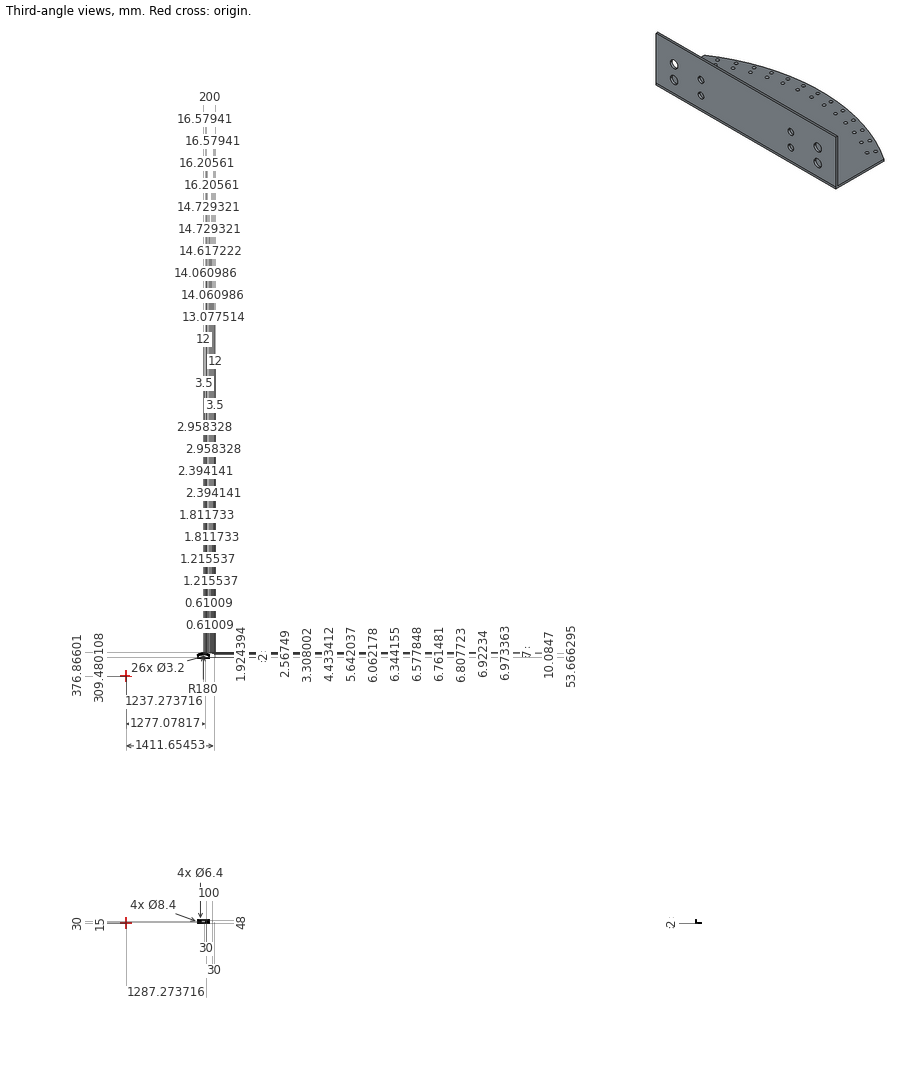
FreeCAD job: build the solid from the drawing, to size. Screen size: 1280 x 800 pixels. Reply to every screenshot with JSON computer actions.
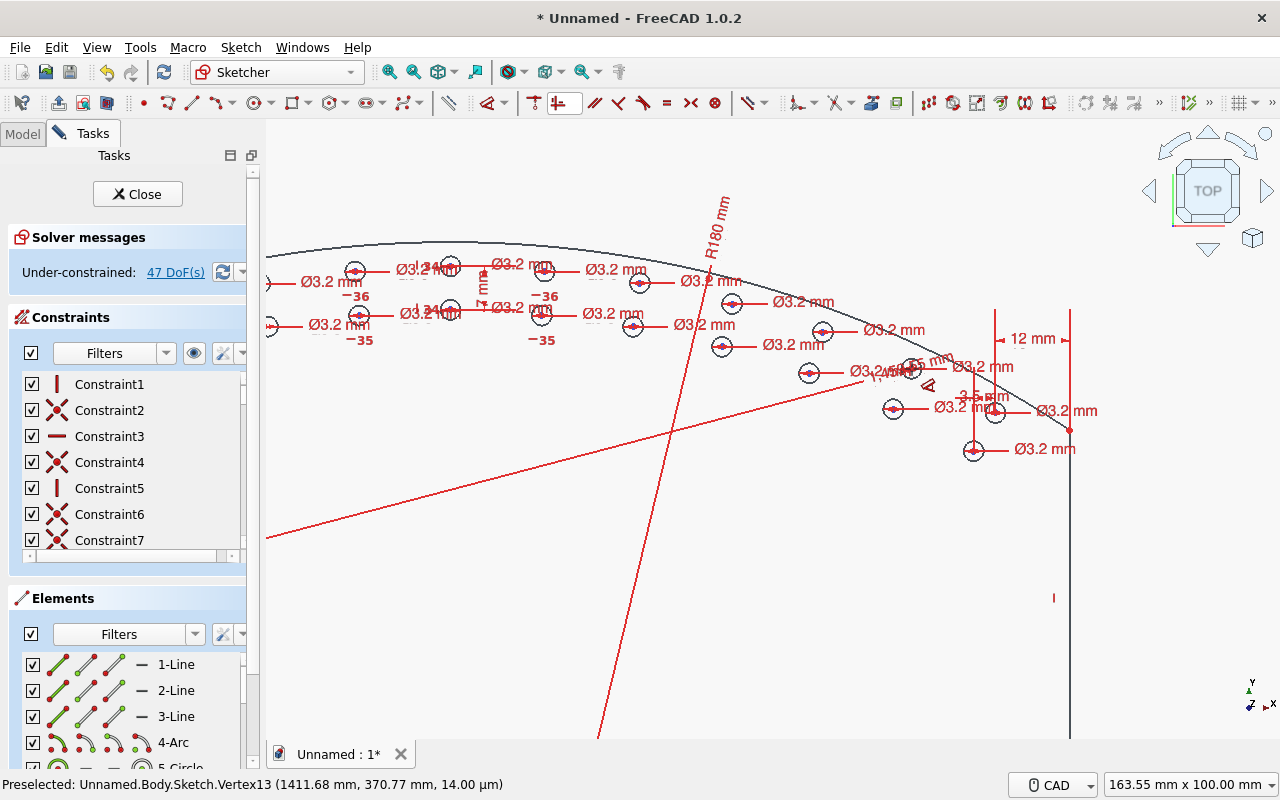
{"action": "left_click", "coordinate": [633, 327]}
{"action": "left_click", "coordinate": [946, 338]}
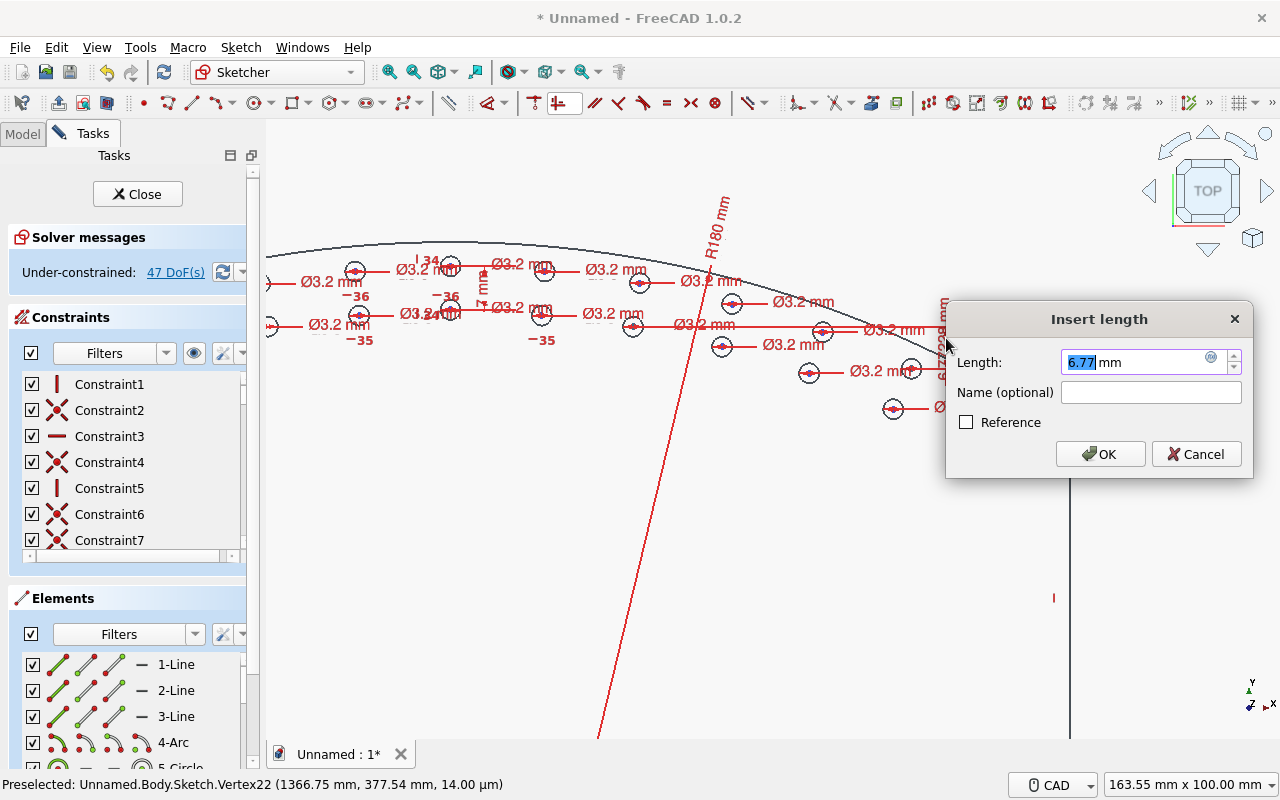
{"action": "type", "text": "6.92234"}
{"action": "key", "text": "Return"}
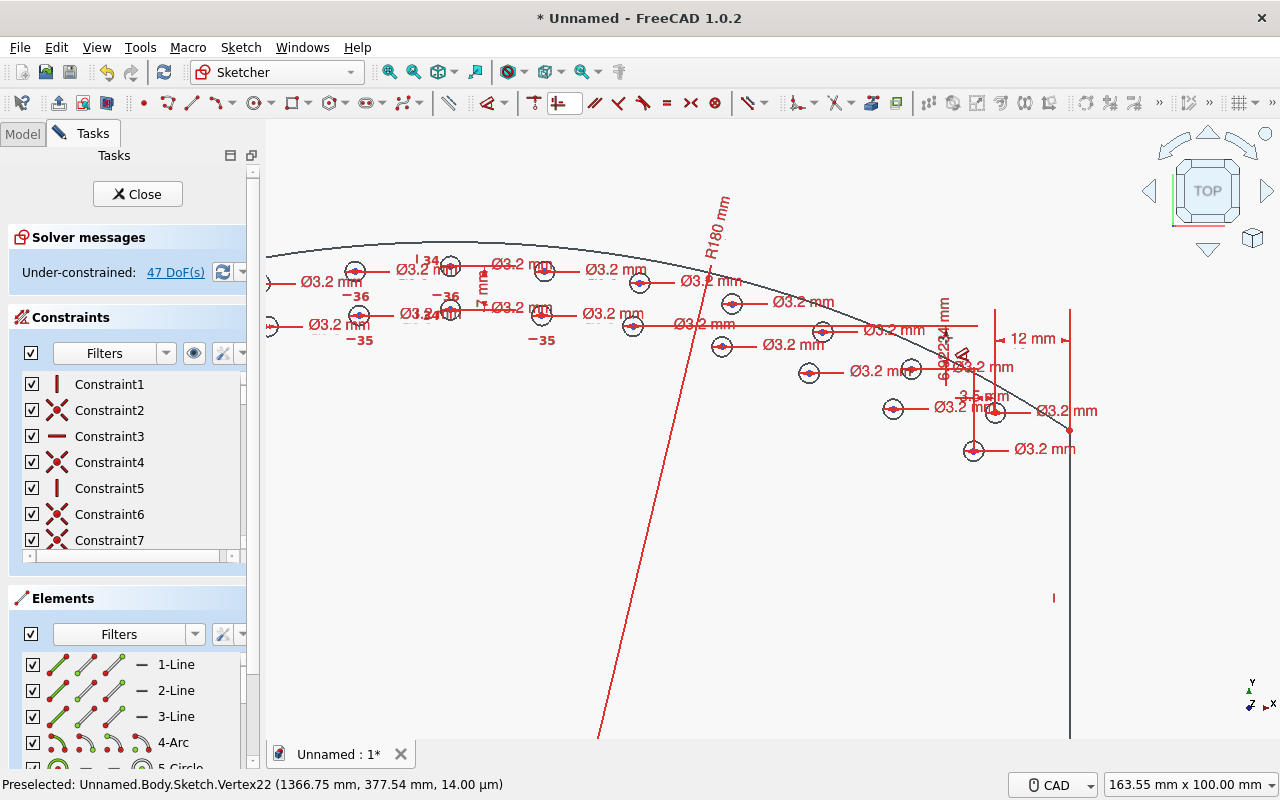
{"action": "scroll", "coordinate": [633, 326], "scroll_direction": "up", "scroll_amount": 5}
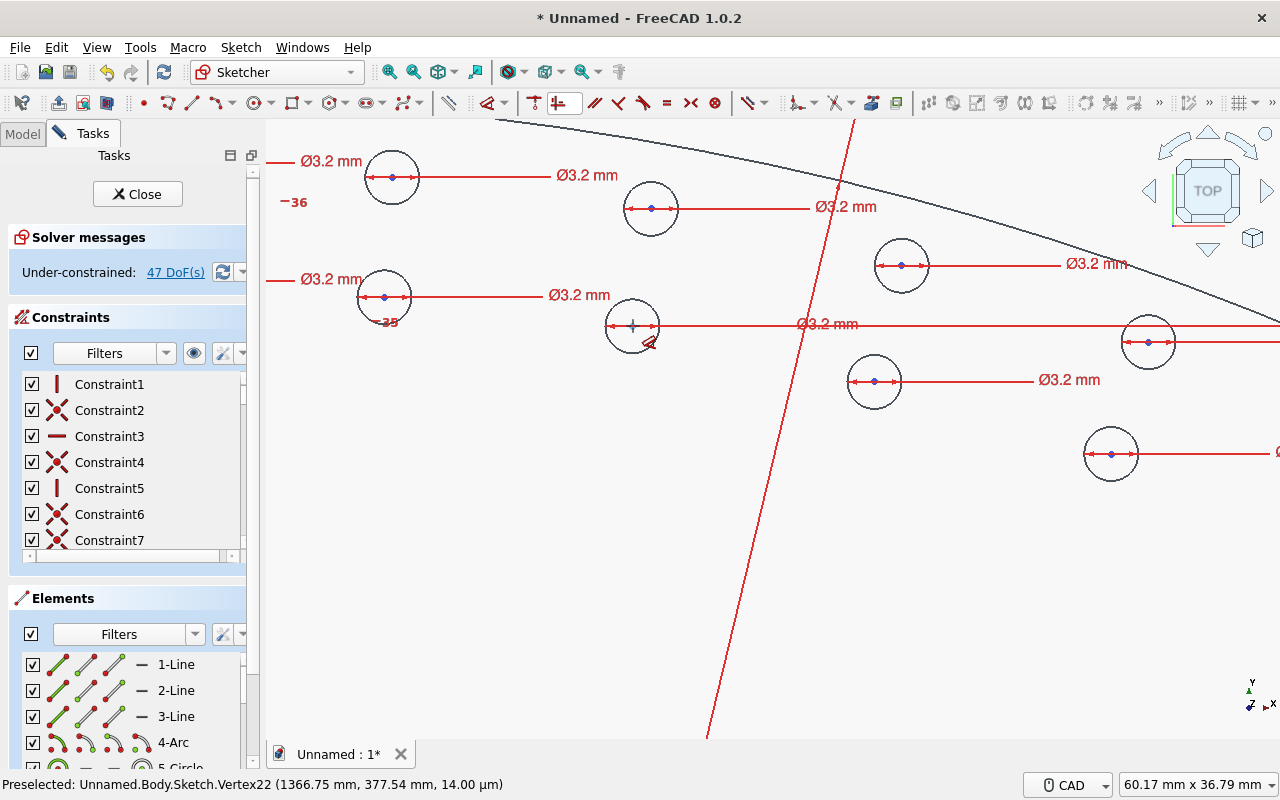
{"action": "left_click", "coordinate": [632, 326]}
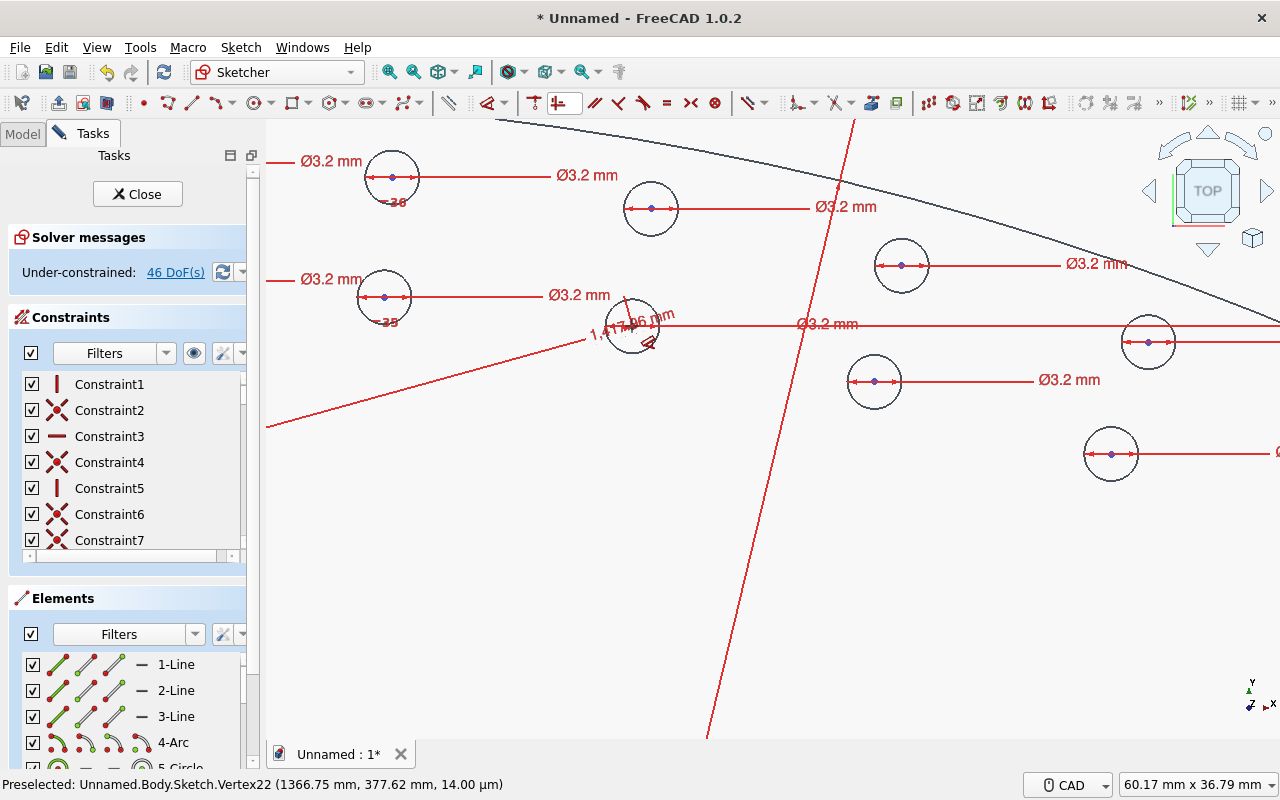
{"action": "scroll", "coordinate": [817, 355], "scroll_direction": "down", "scroll_amount": 9}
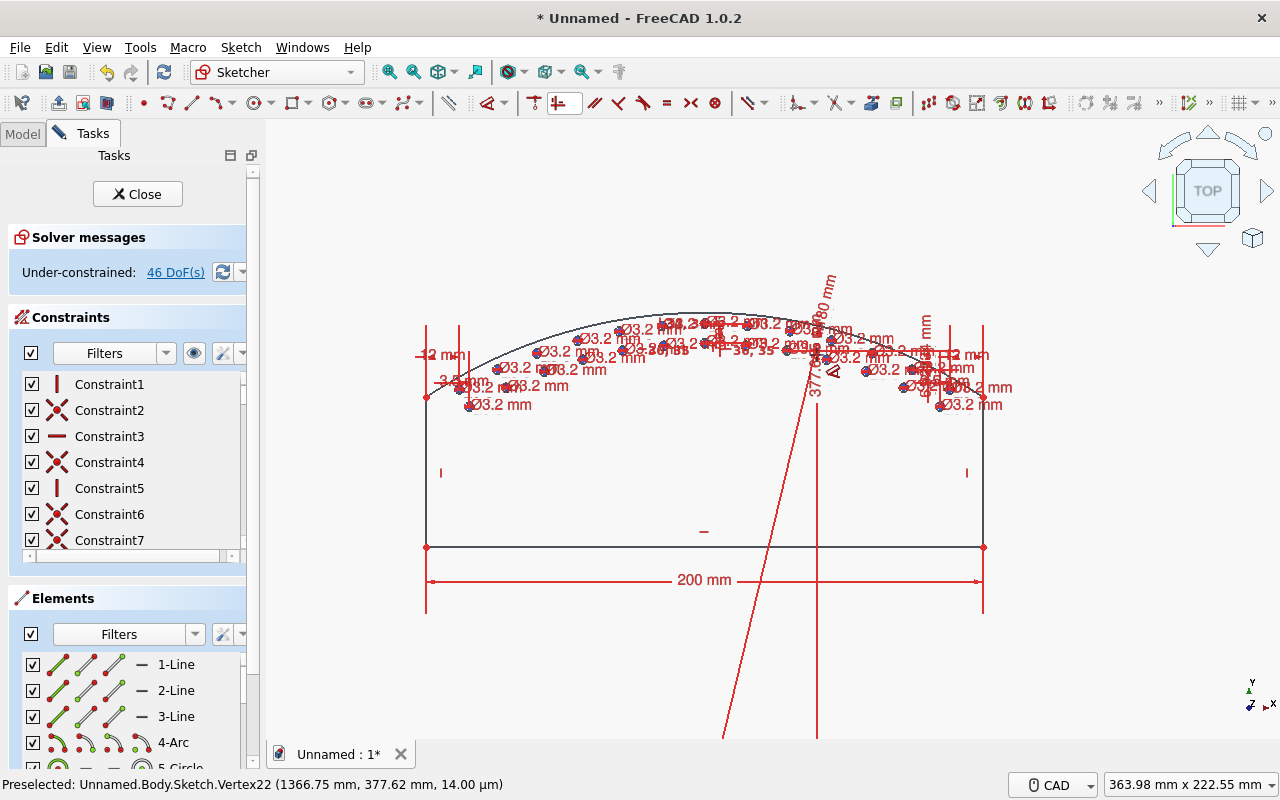
{"action": "scroll", "coordinate": [705, 343], "scroll_direction": "up", "scroll_amount": 9}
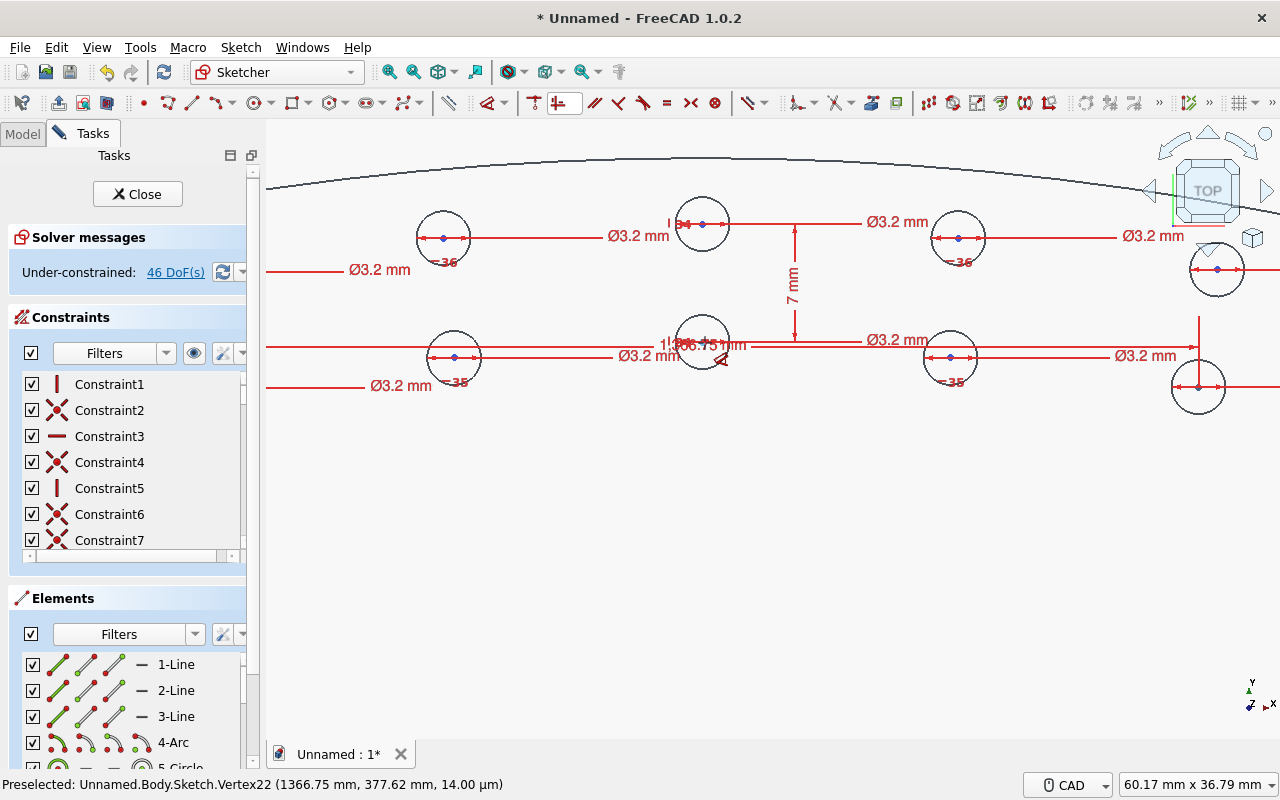
{"action": "left_click", "coordinate": [702, 342]}
{"action": "left_click", "coordinate": [668, 365]}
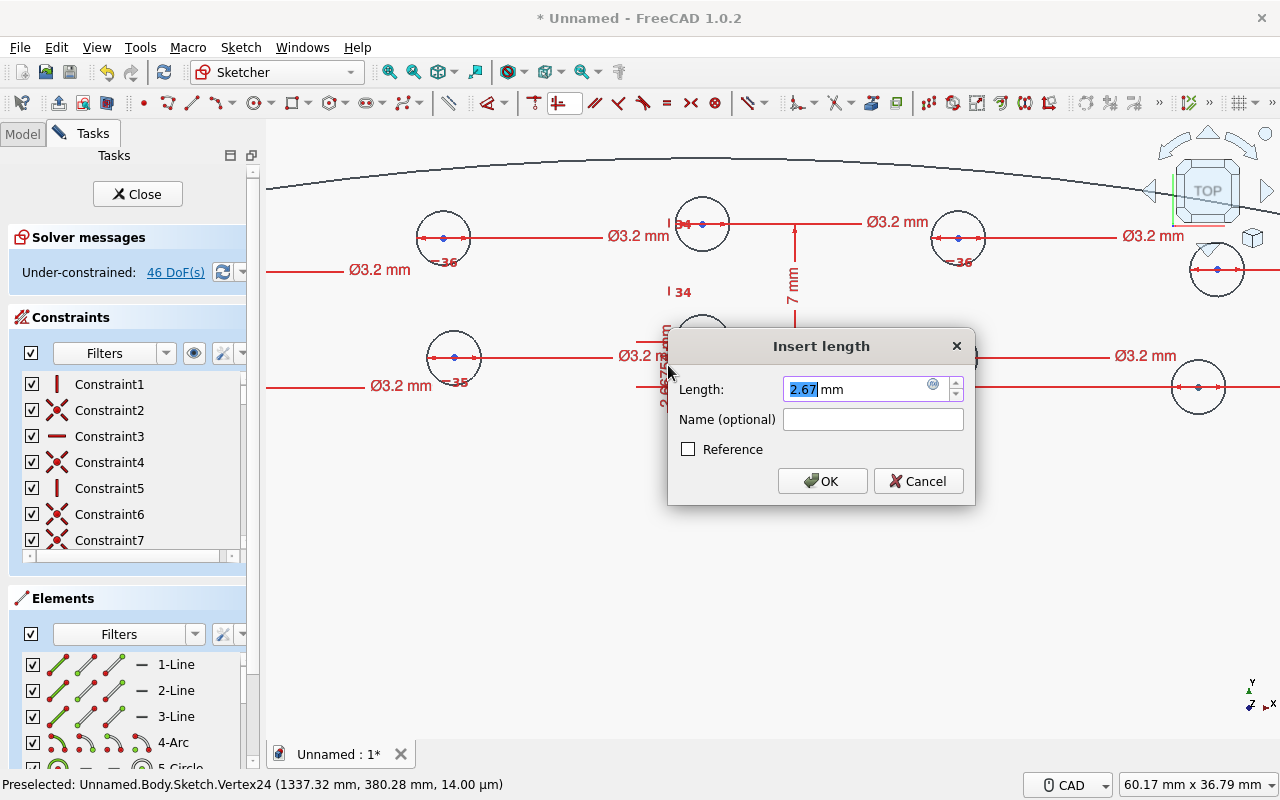
{"action": "type", "text": "2.56749"}
{"action": "key", "text": "Return"}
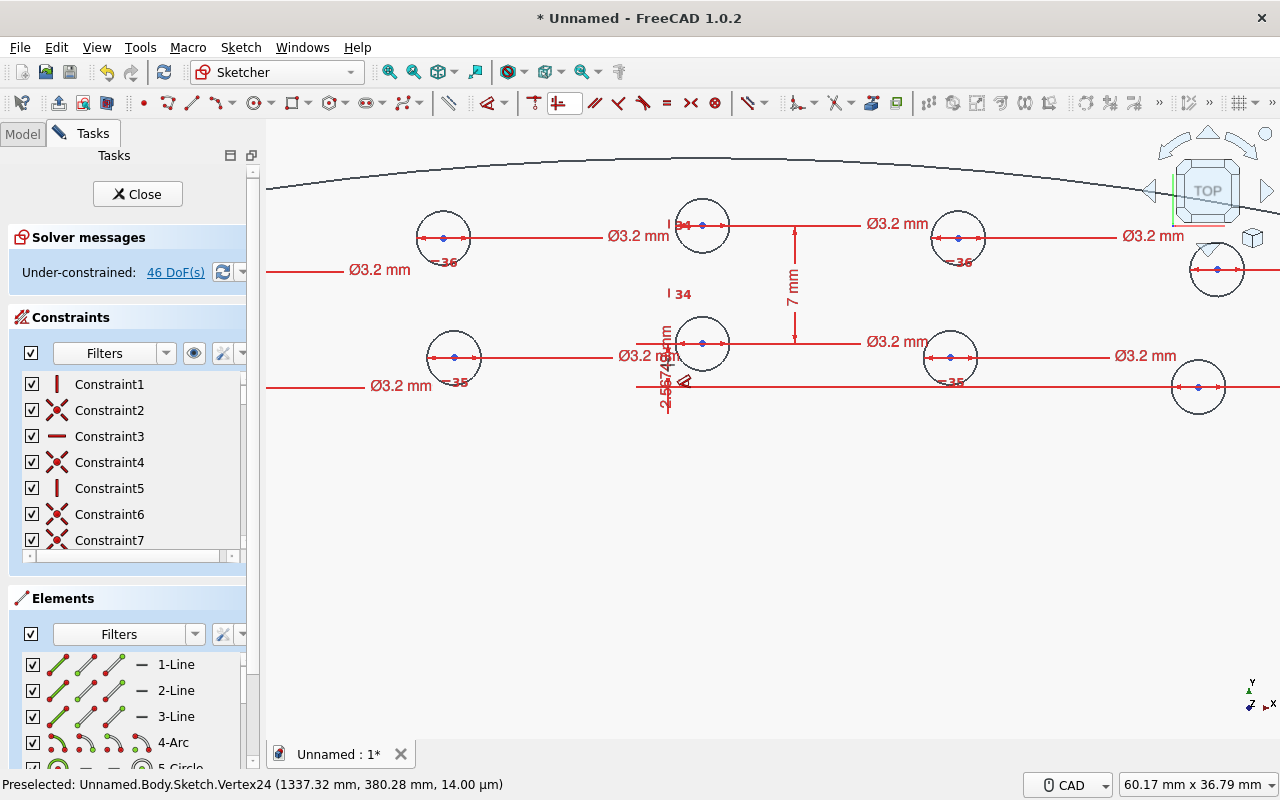
{"action": "scroll", "coordinate": [705, 343], "scroll_direction": "down", "scroll_amount": 9}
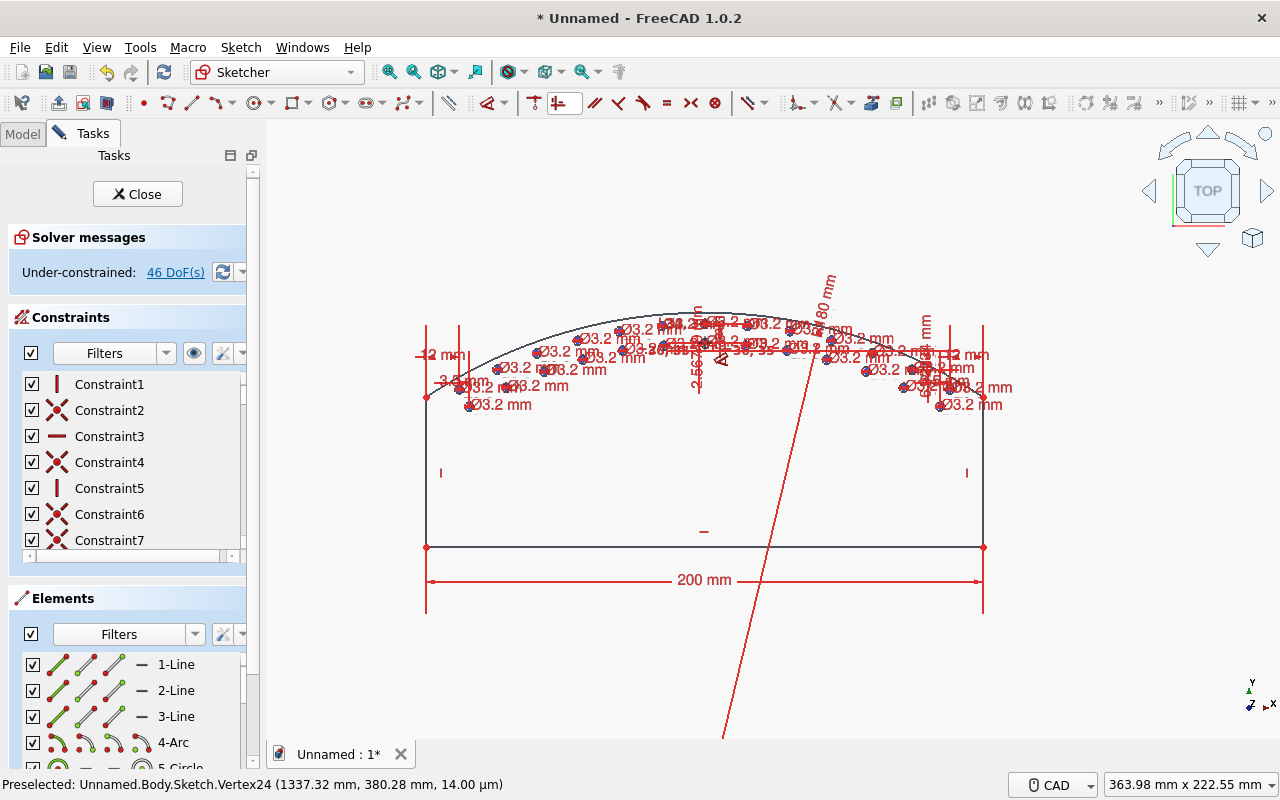
{"action": "scroll", "coordinate": [827, 360], "scroll_direction": "up", "scroll_amount": 2}